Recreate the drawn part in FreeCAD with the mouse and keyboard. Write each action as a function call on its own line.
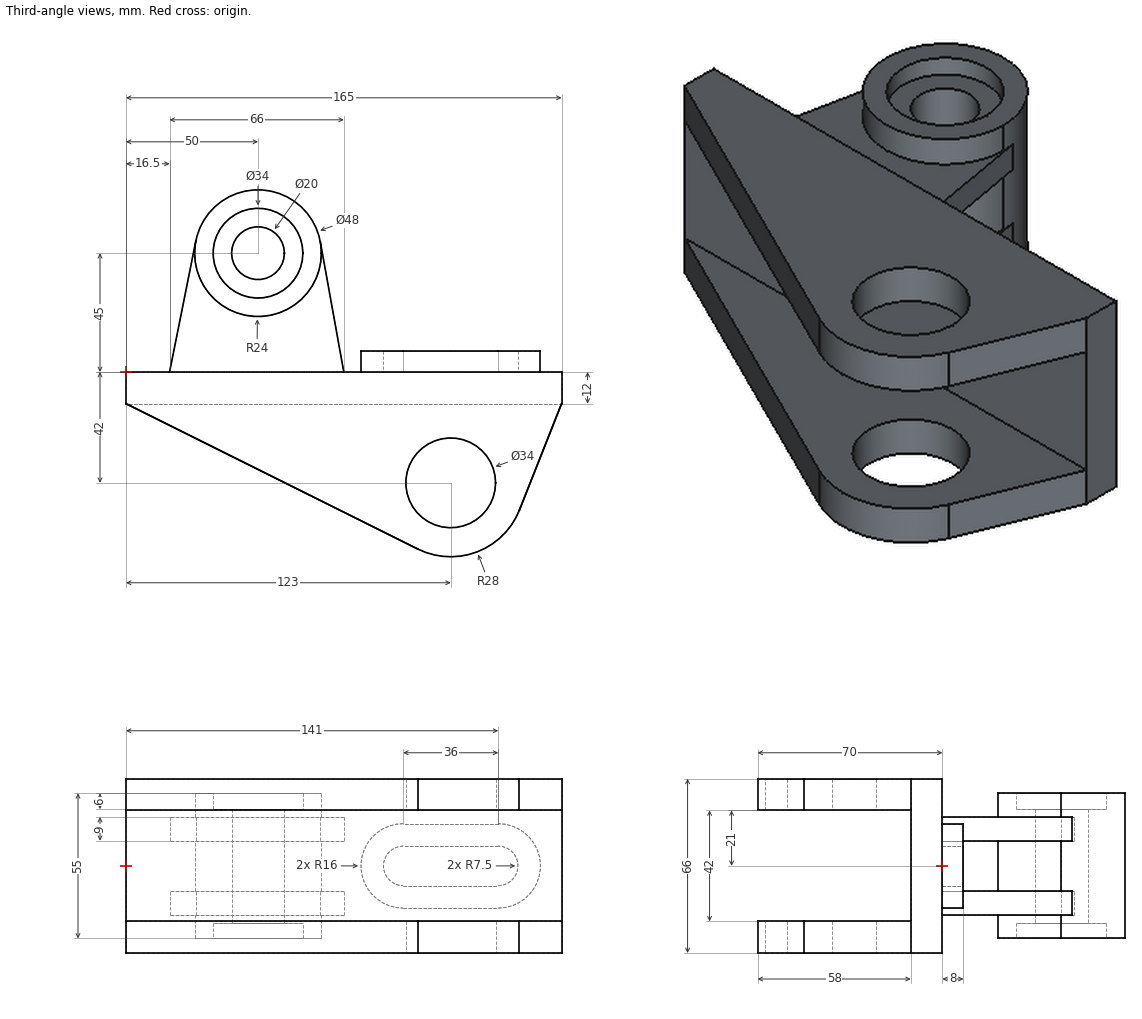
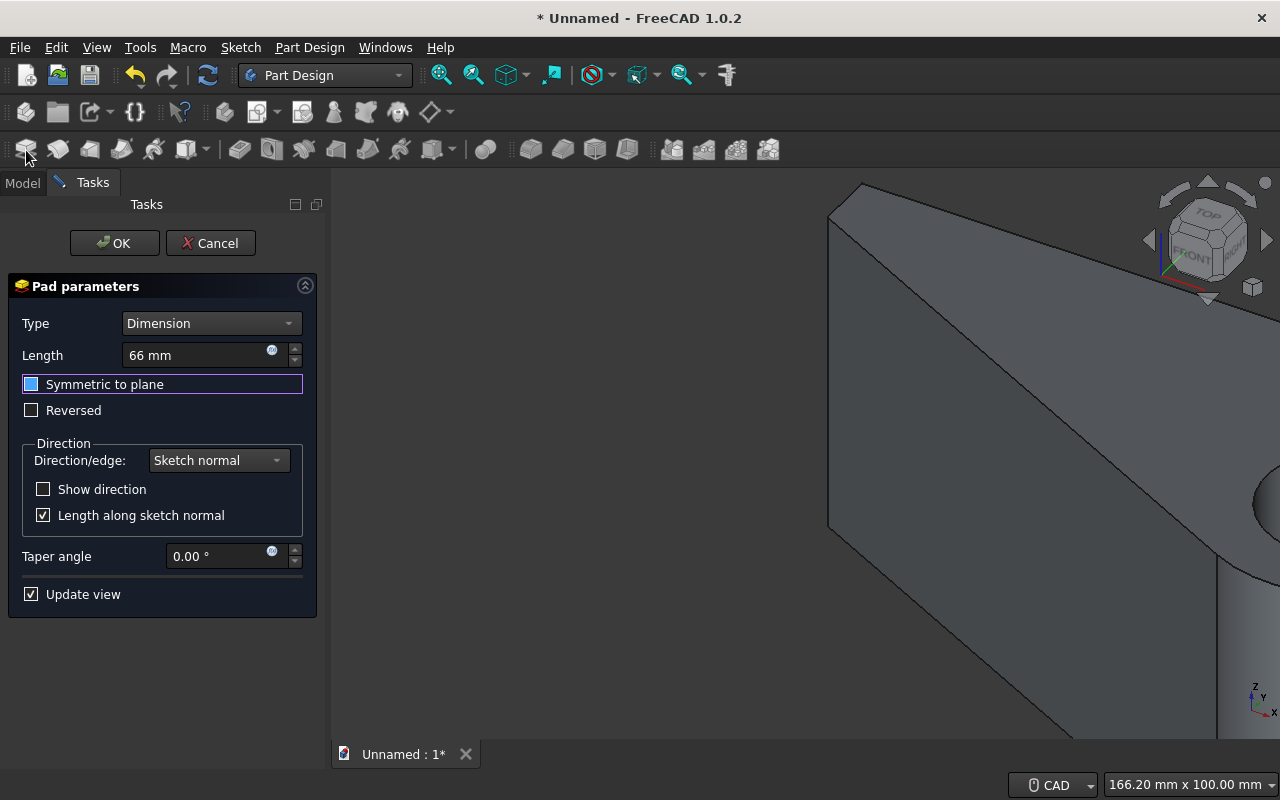
click(30, 384)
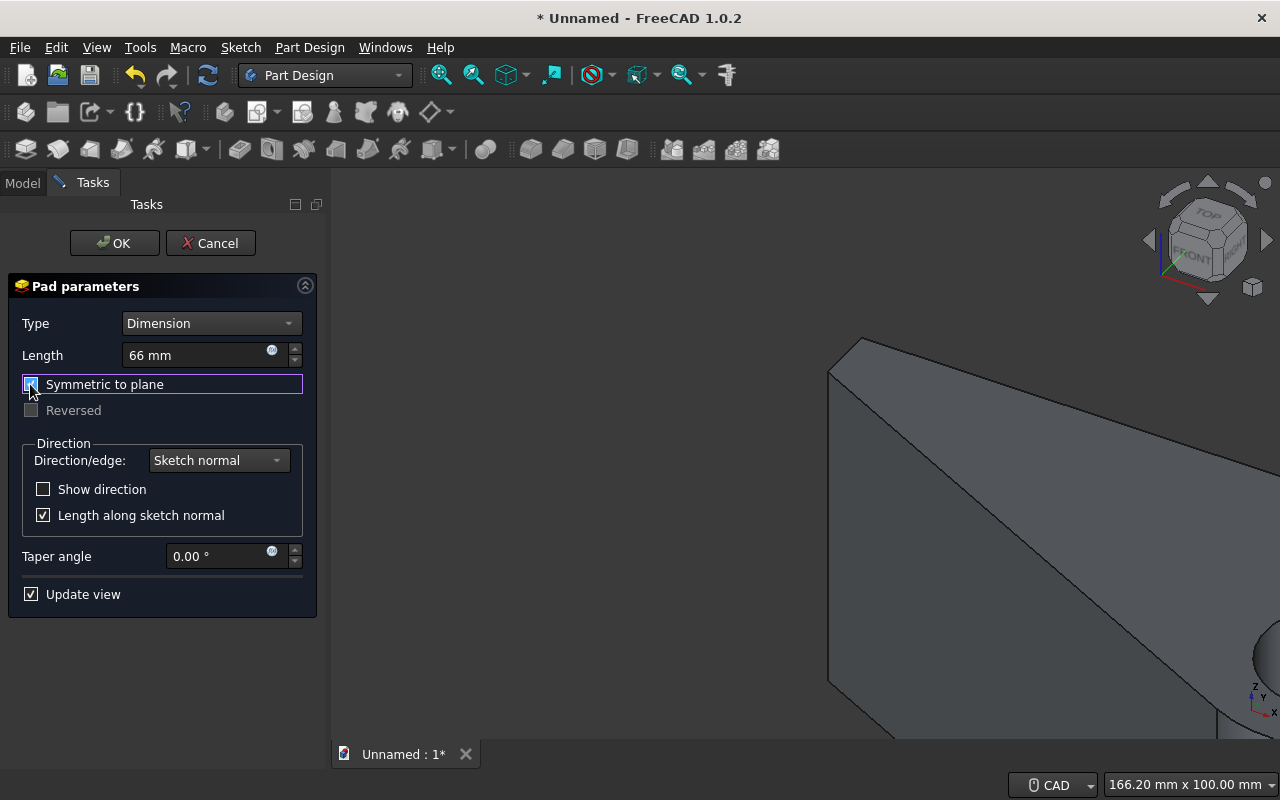
click(115, 243)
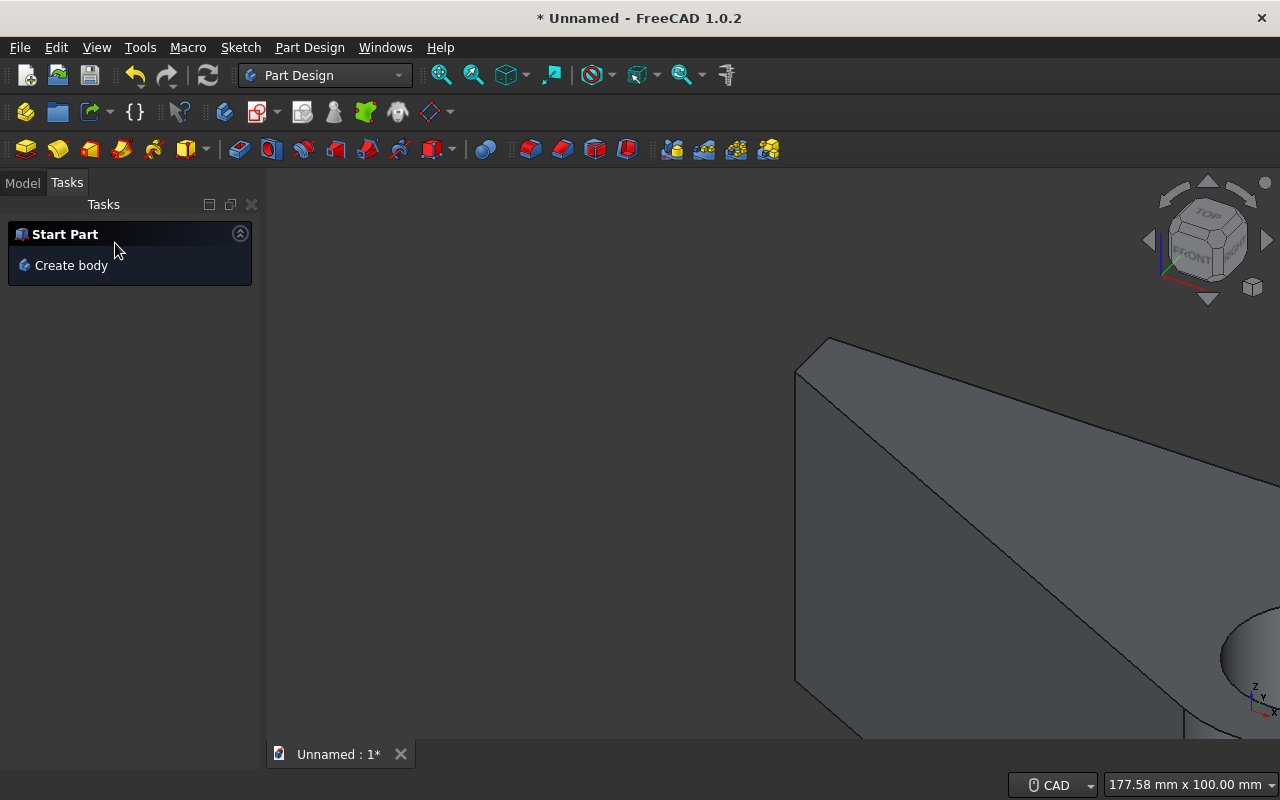
click(442, 76)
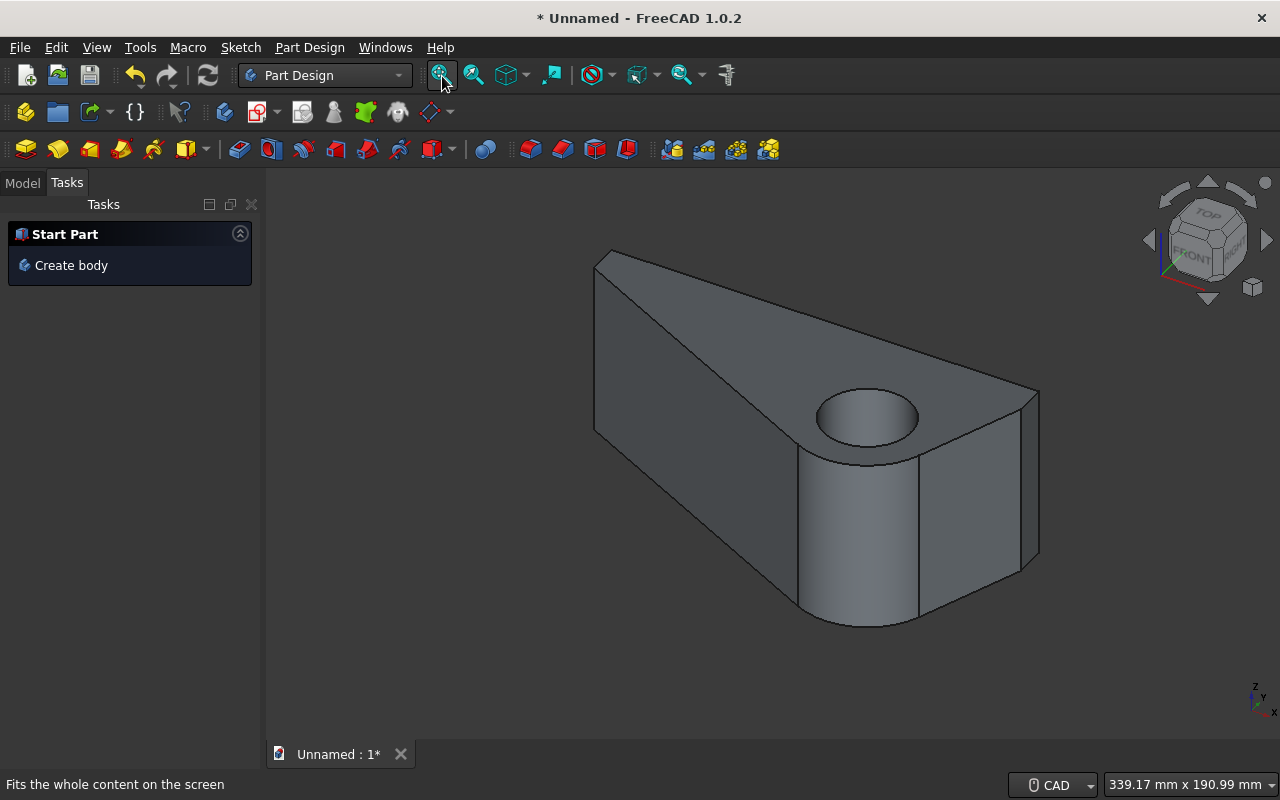
click(1030, 434)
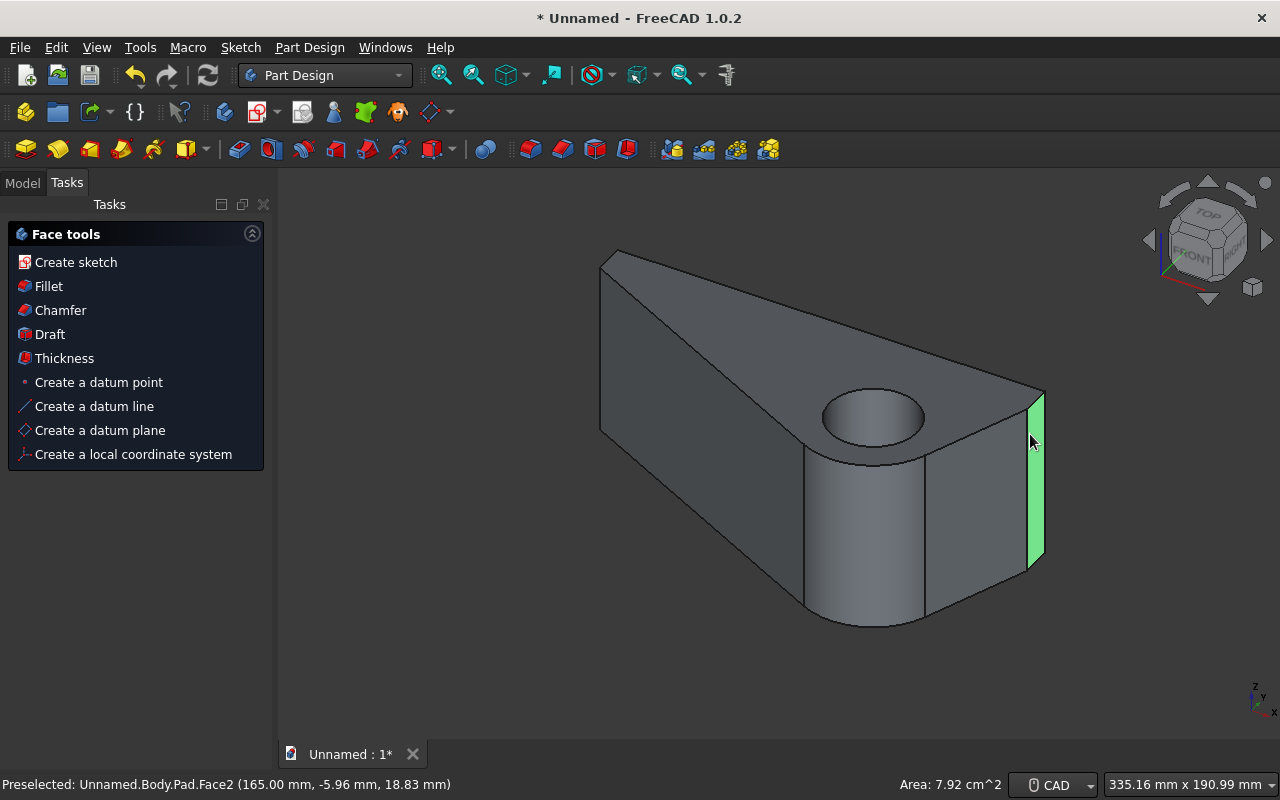
click(258, 112)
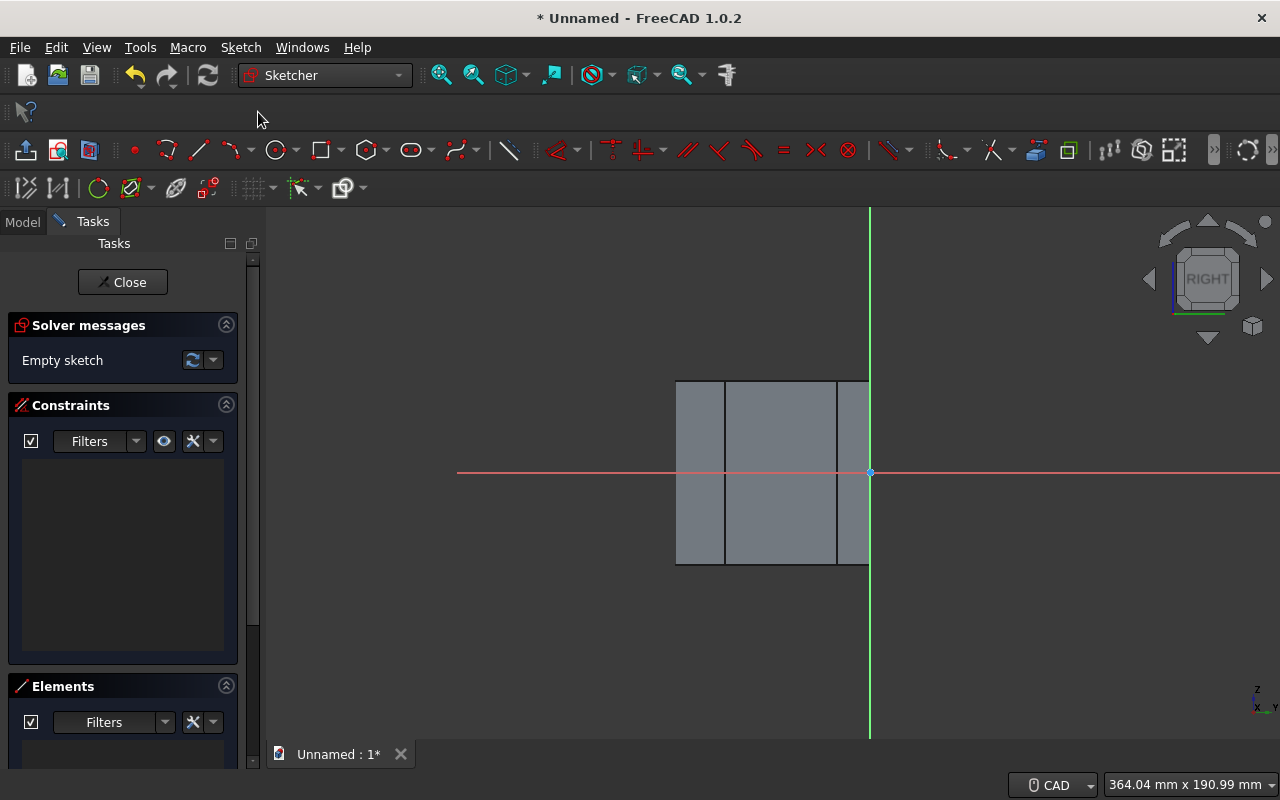
scroll(813, 473, up, 5)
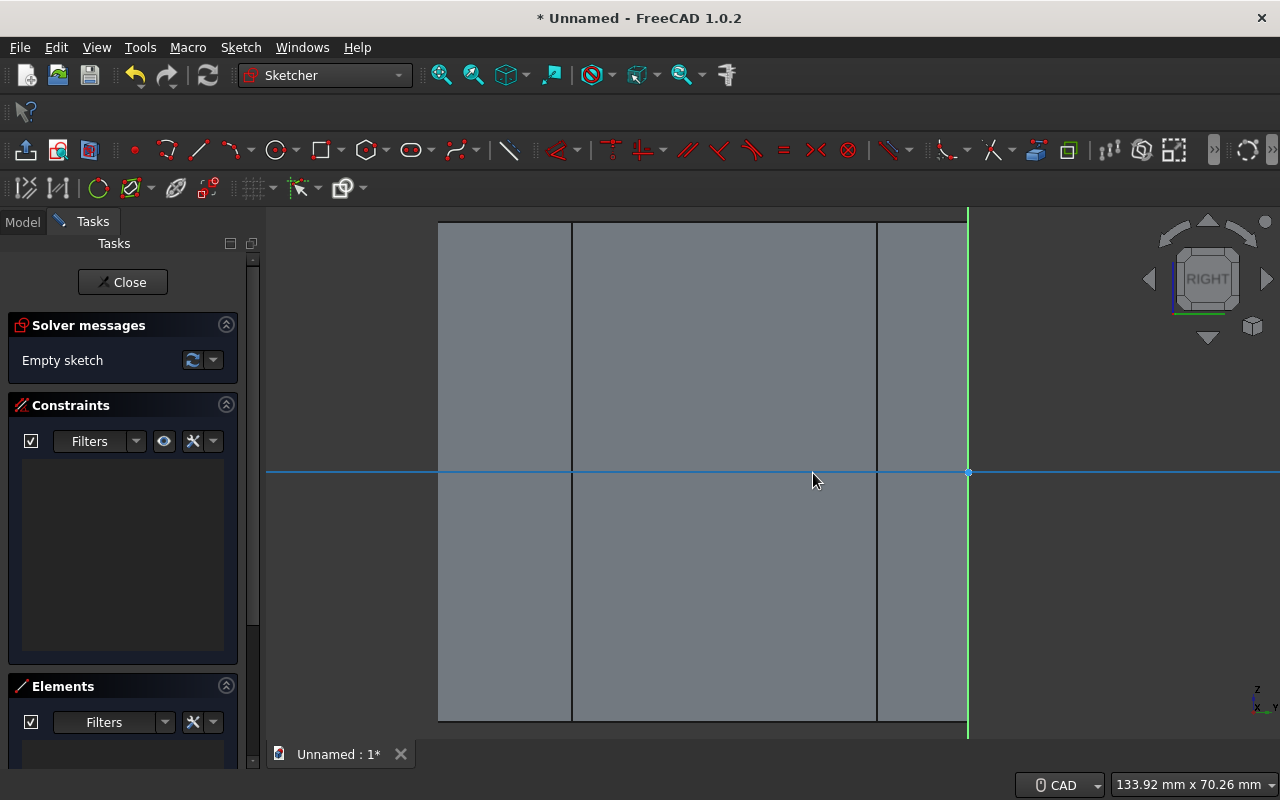
key(g)
key(r)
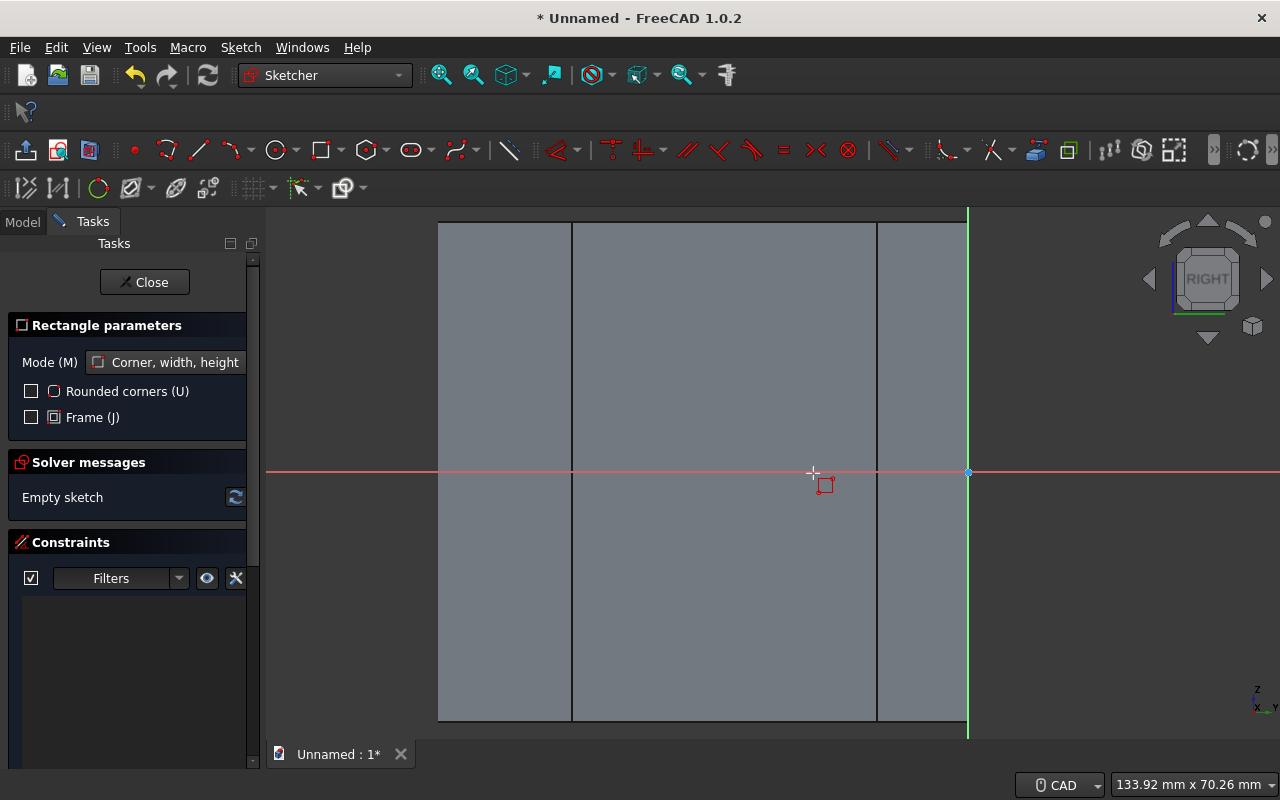
click(438, 313)
move(877, 631)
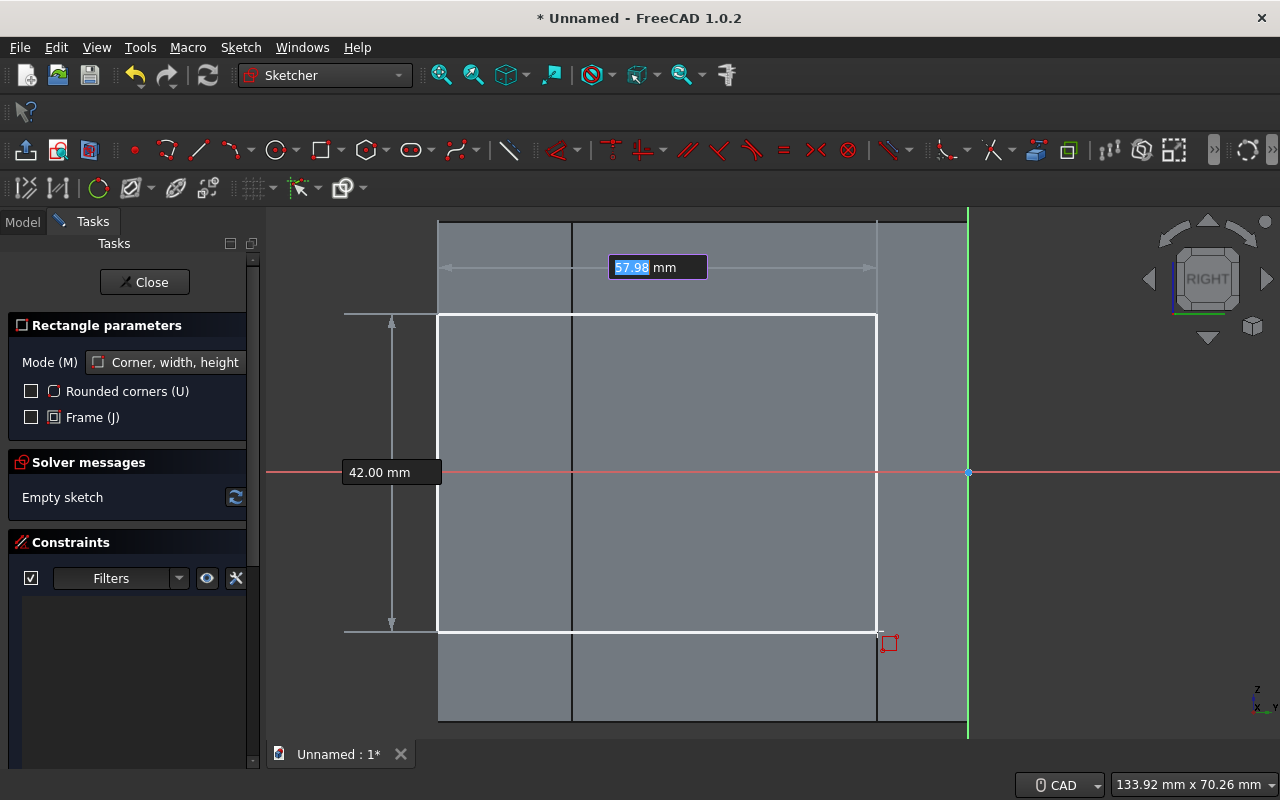
text(58)
key(Tab)
text(42)
key(Return)
key(Escape)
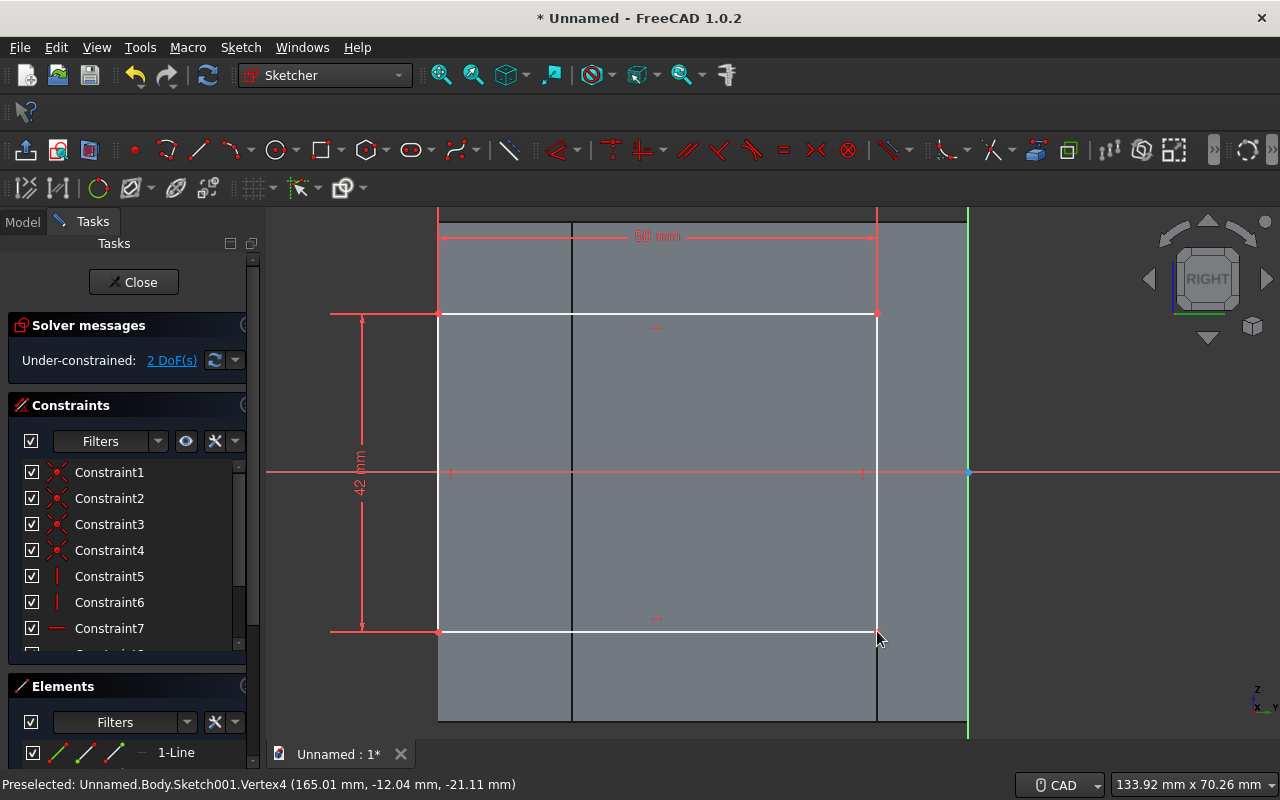
key(d)